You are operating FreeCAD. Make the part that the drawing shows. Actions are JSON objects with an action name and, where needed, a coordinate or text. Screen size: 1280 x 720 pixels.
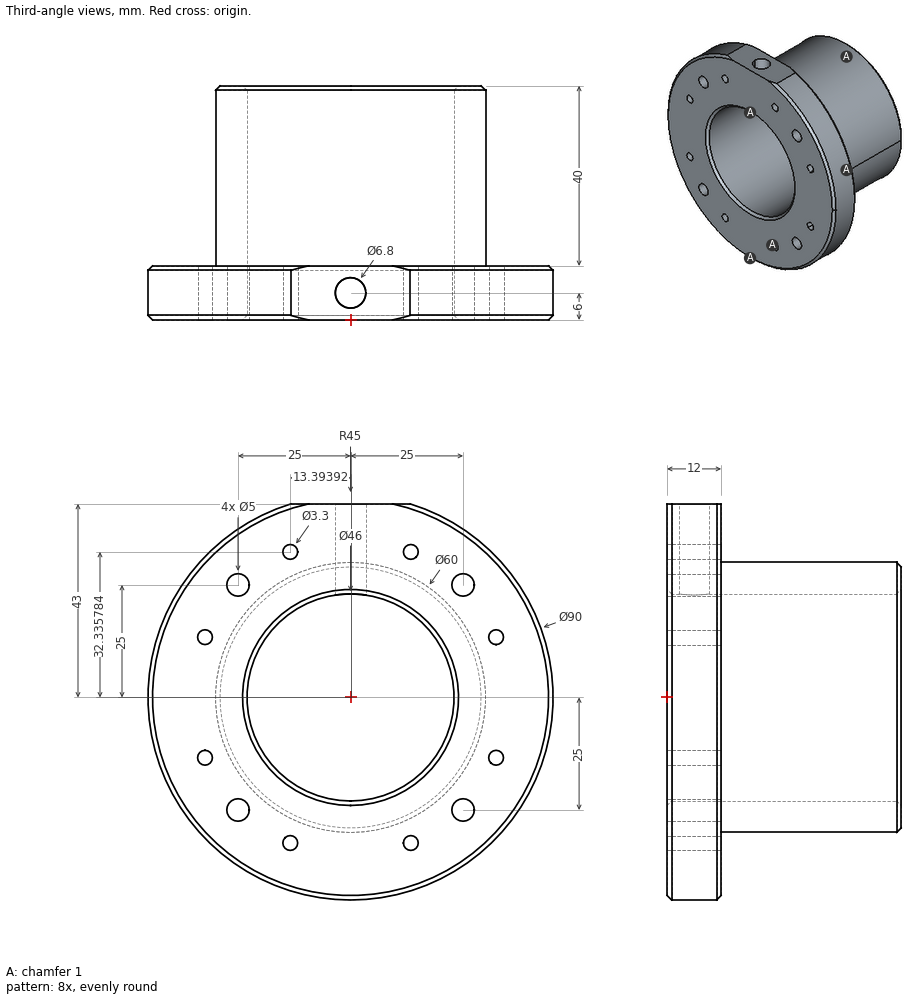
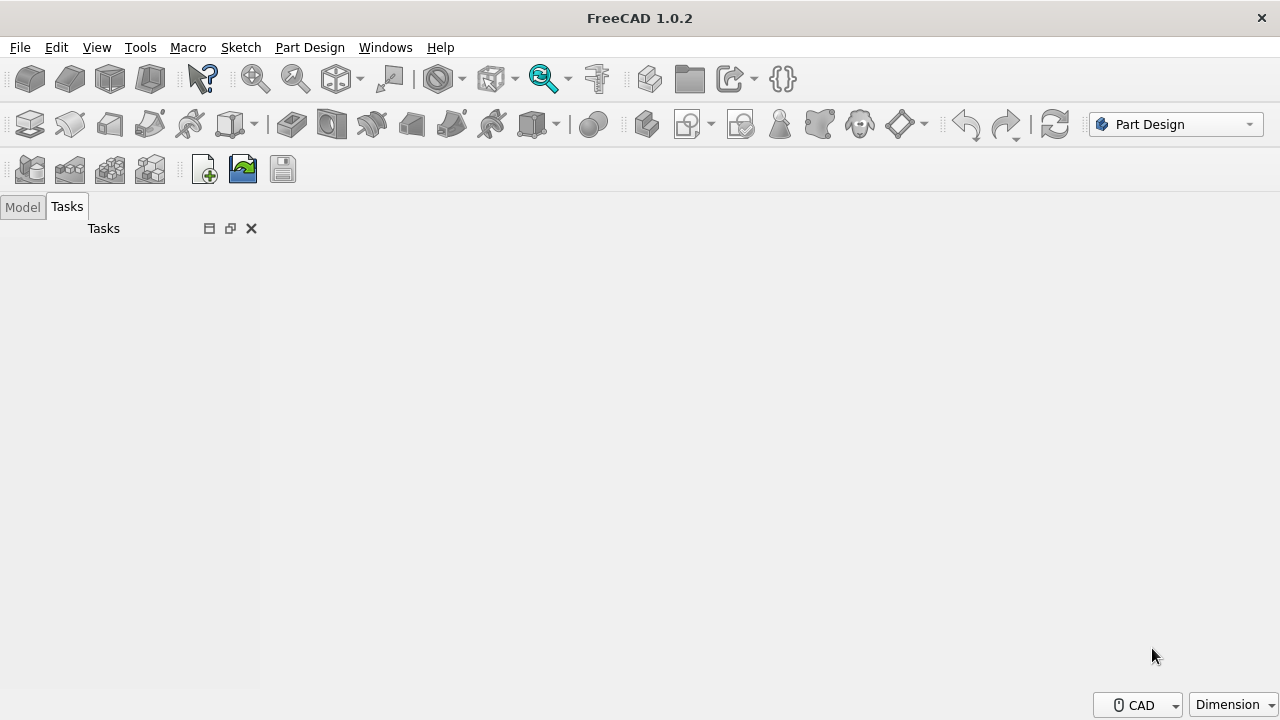
{"action": "key", "text": "ctrl+n"}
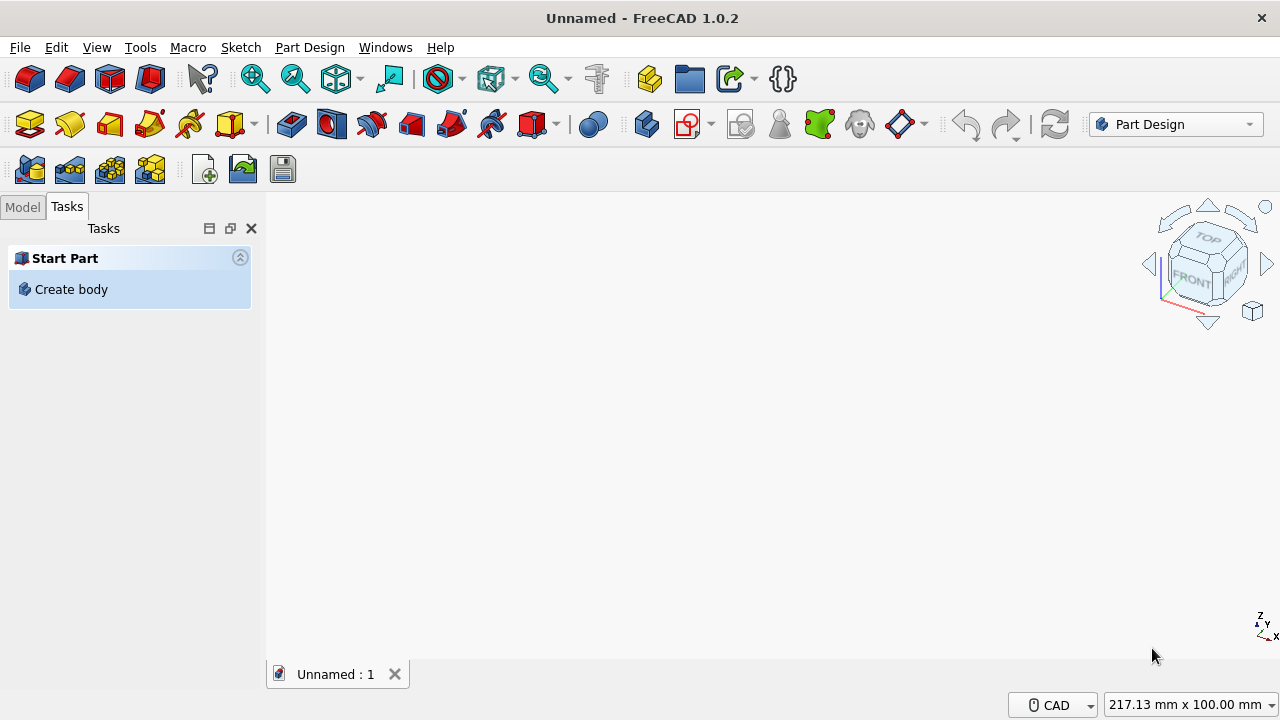
{"action": "left_click", "coordinate": [688, 124]}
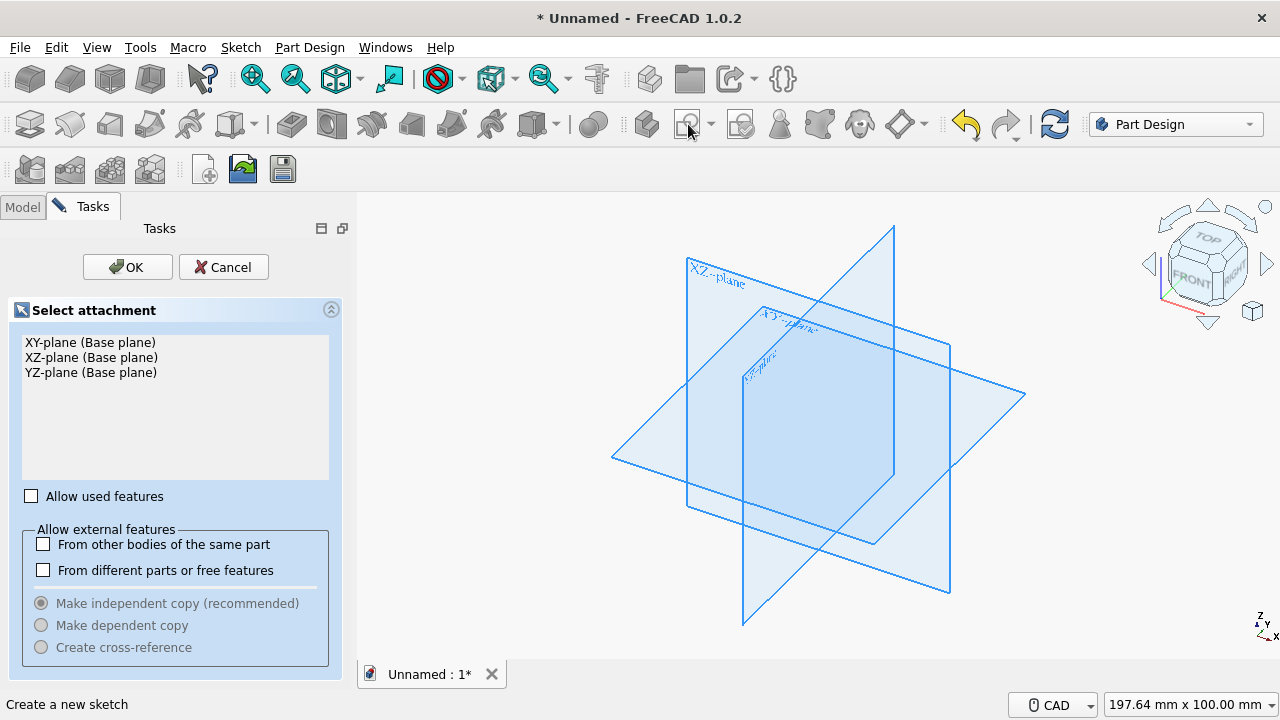
{"action": "left_click", "coordinate": [82, 358]}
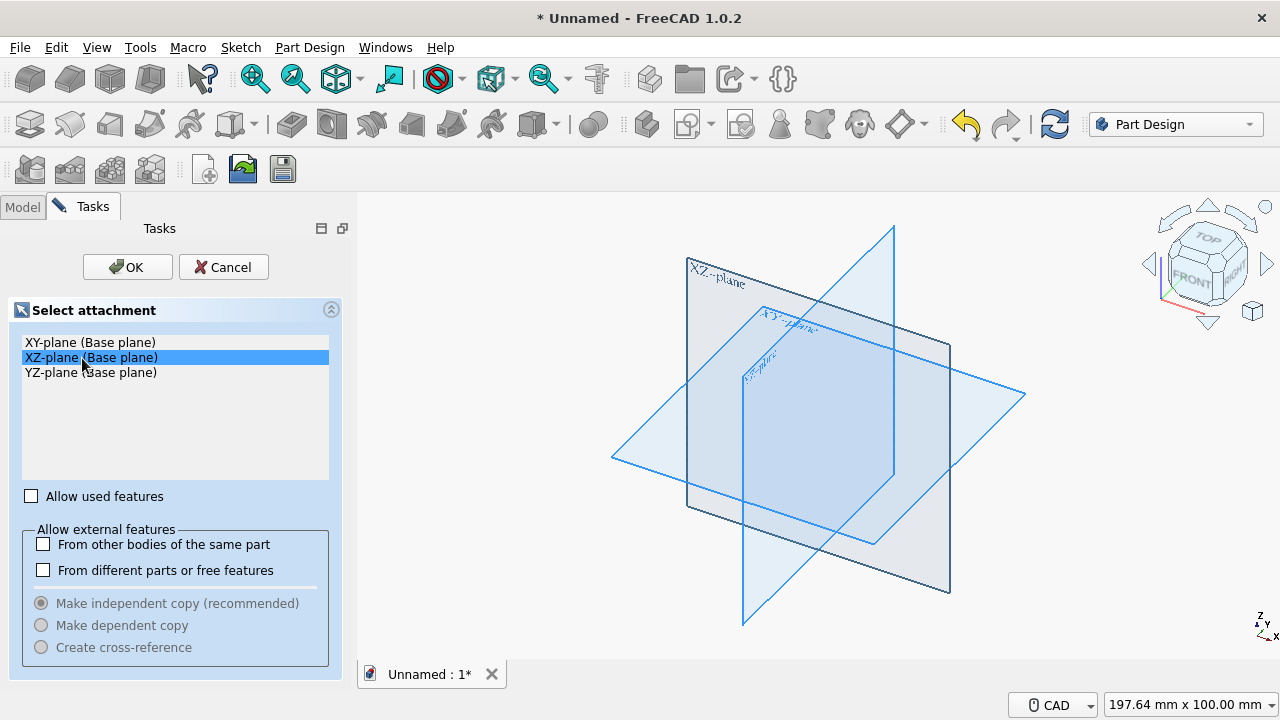
{"action": "left_click", "coordinate": [128, 267]}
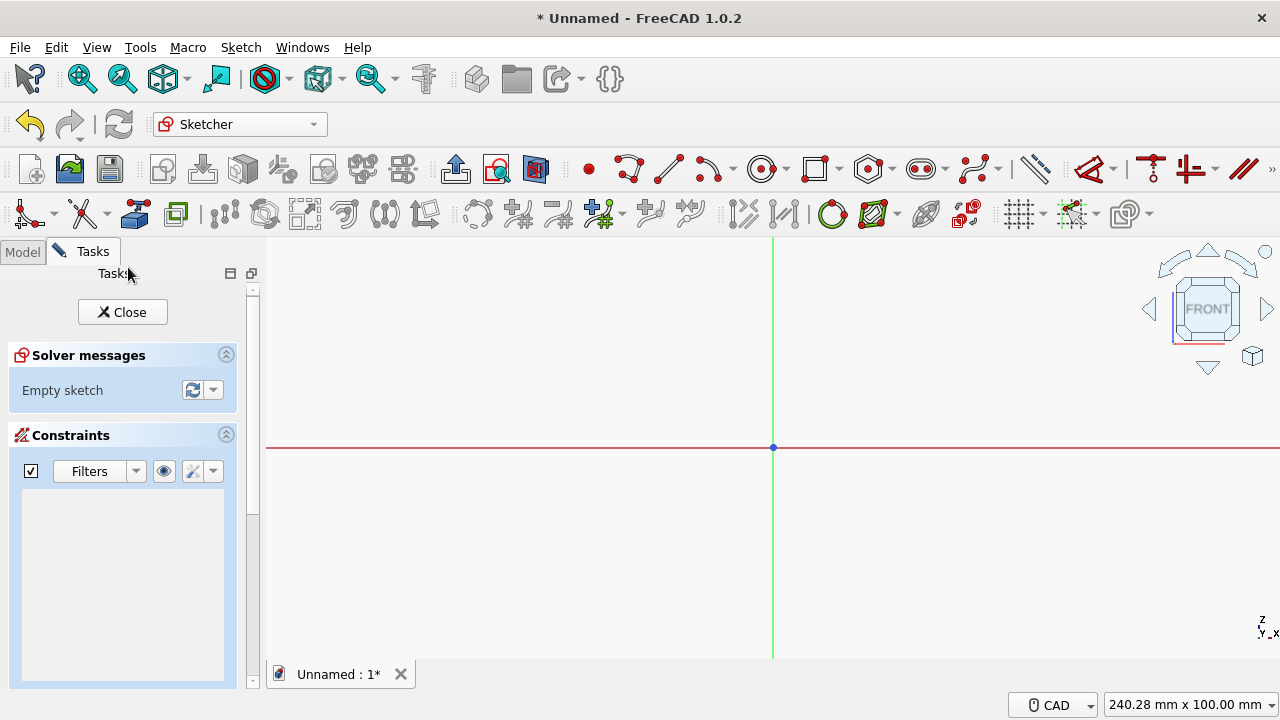
{"action": "scroll", "coordinate": [565, 448], "scroll_direction": "down", "scroll_amount": 2}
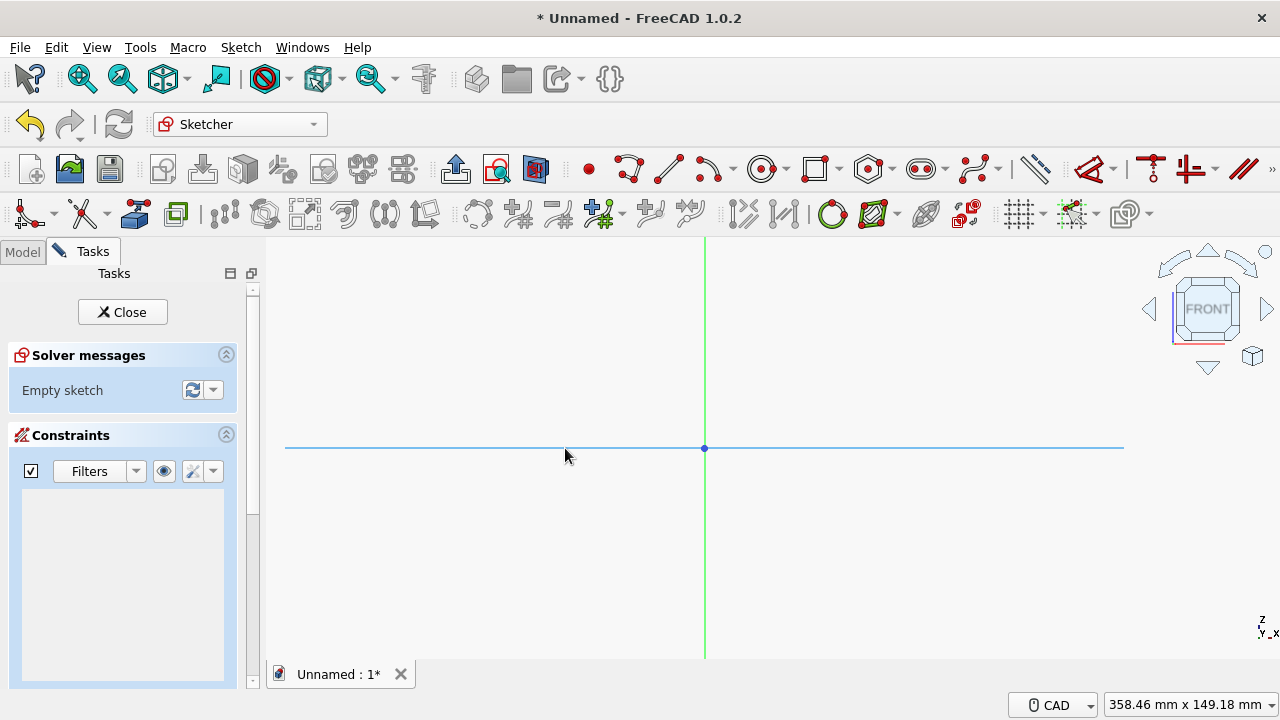
{"action": "key", "text": "g c"}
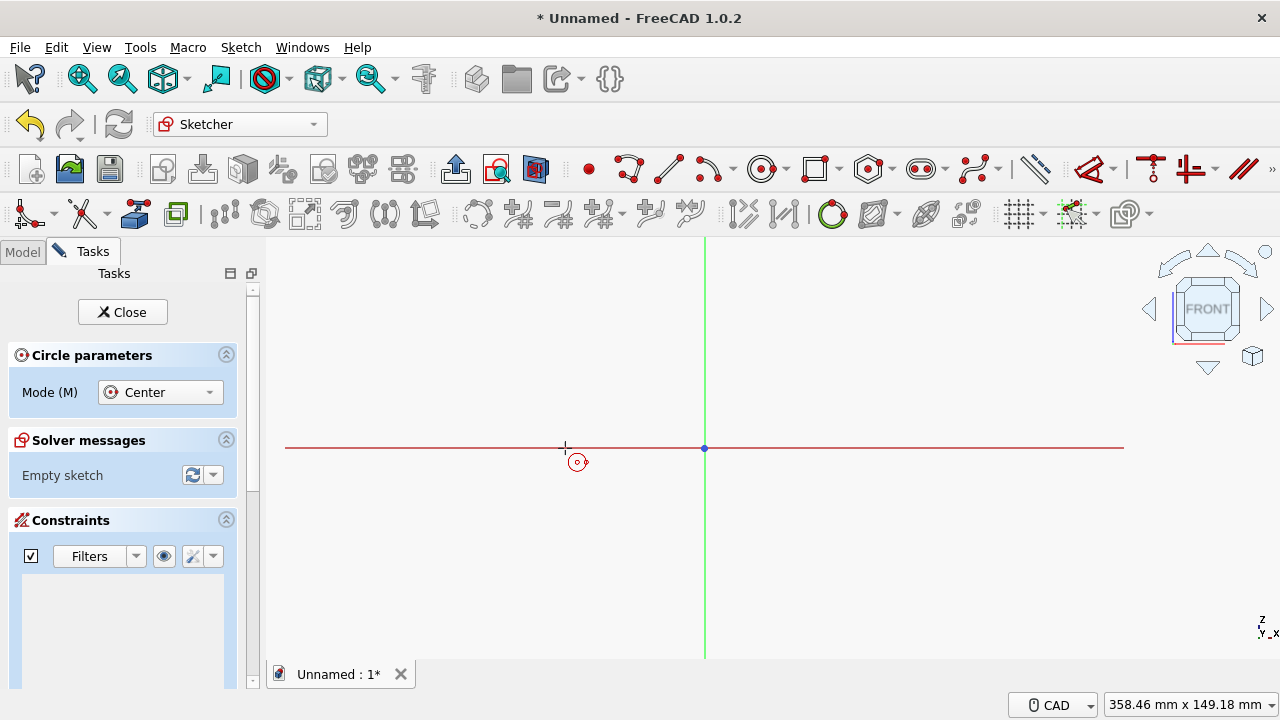
{"action": "left_click", "coordinate": [705, 448]}
{"action": "left_click", "coordinate": [795, 358]}
{"action": "key", "text": "Escape"}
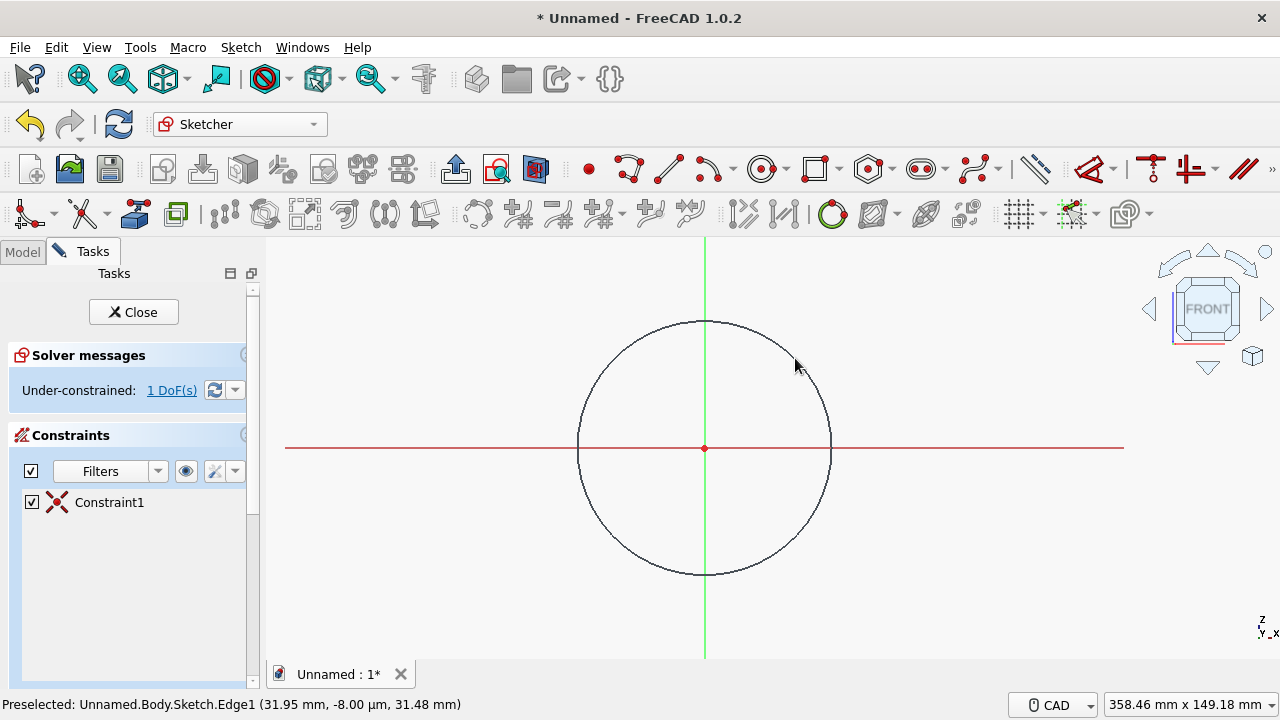
{"action": "key", "text": "d"}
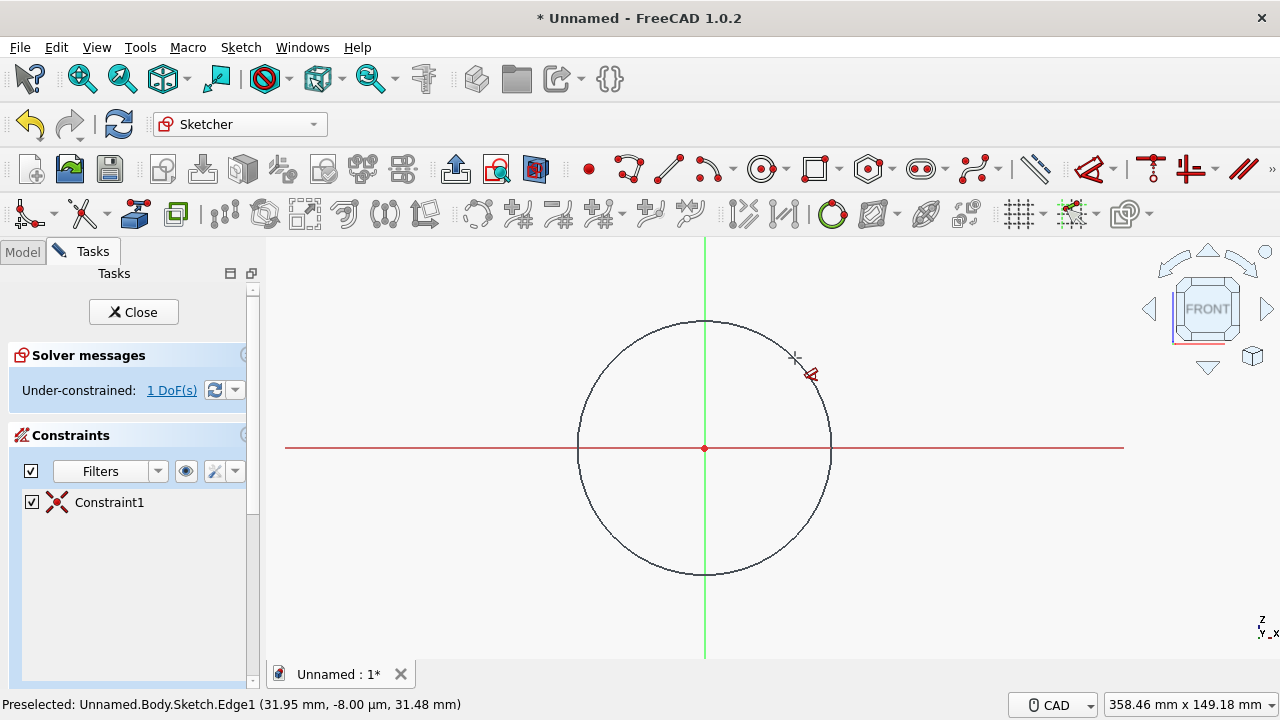
{"action": "left_click", "coordinate": [794, 358]}
{"action": "left_click", "coordinate": [817, 335]}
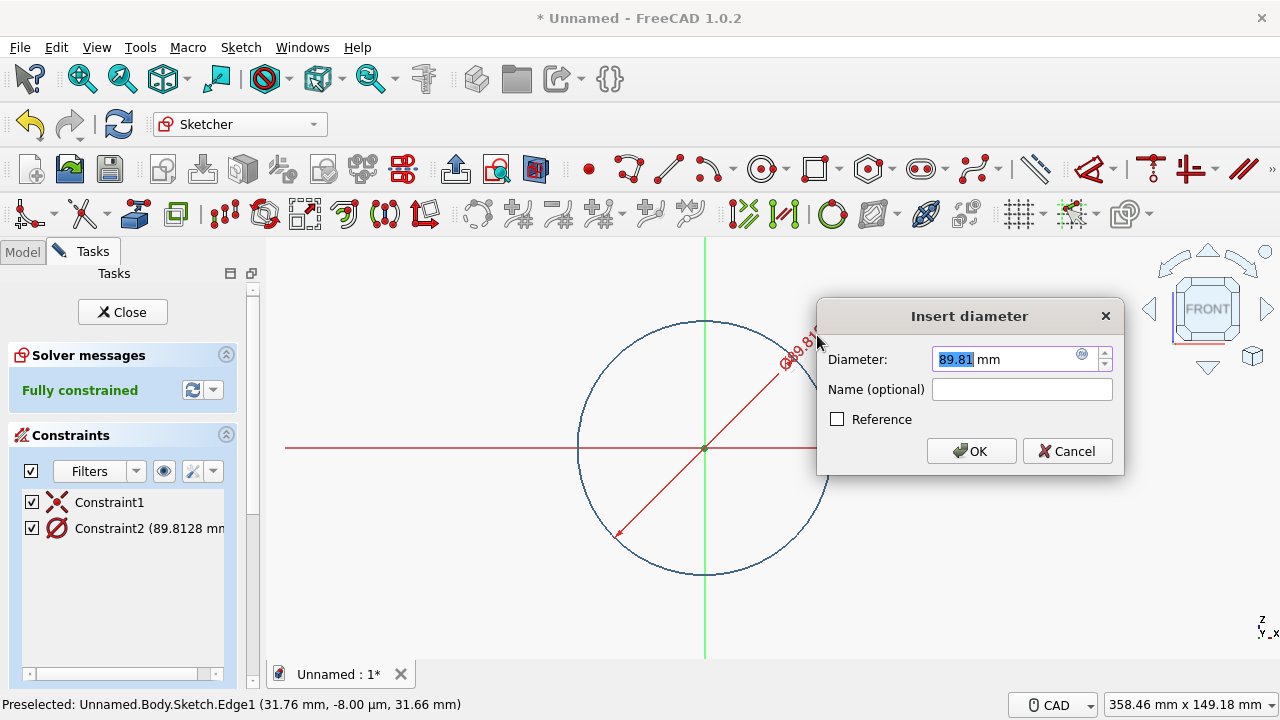
{"action": "type", "text": "90"}
{"action": "key", "text": "Return"}
{"action": "key", "text": "Escape"}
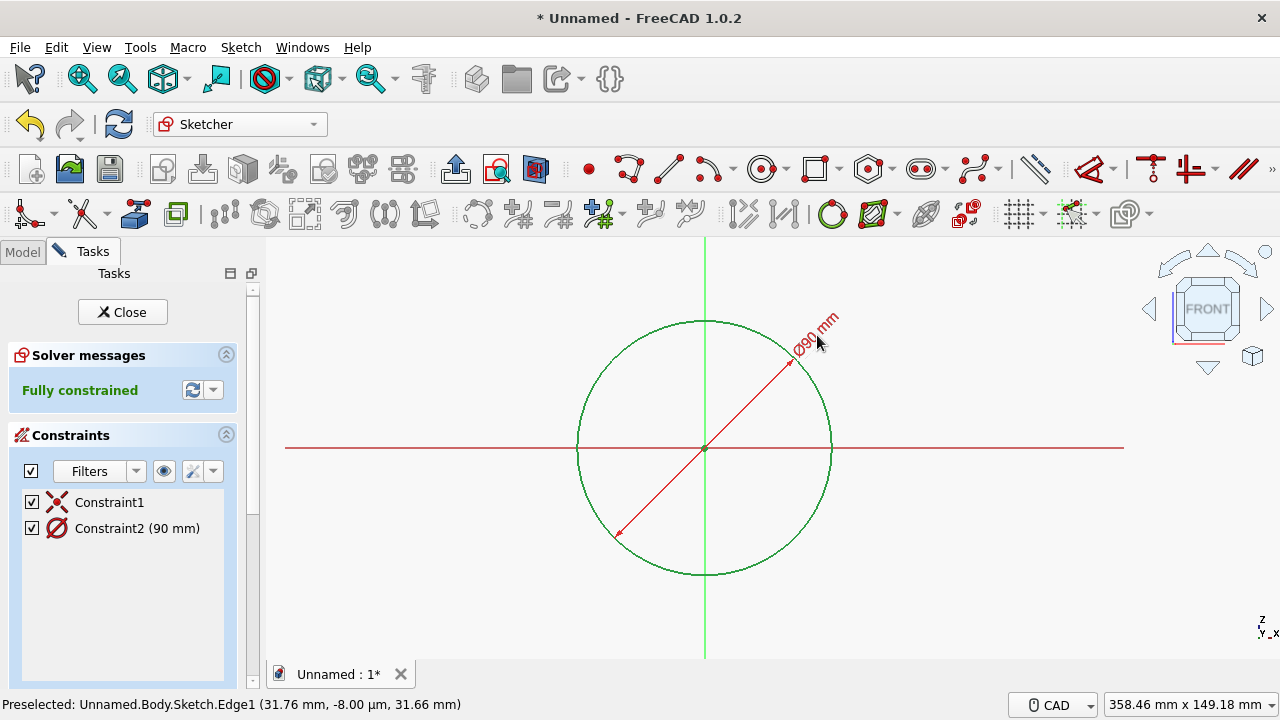
{"action": "left_click", "coordinate": [123, 312]}